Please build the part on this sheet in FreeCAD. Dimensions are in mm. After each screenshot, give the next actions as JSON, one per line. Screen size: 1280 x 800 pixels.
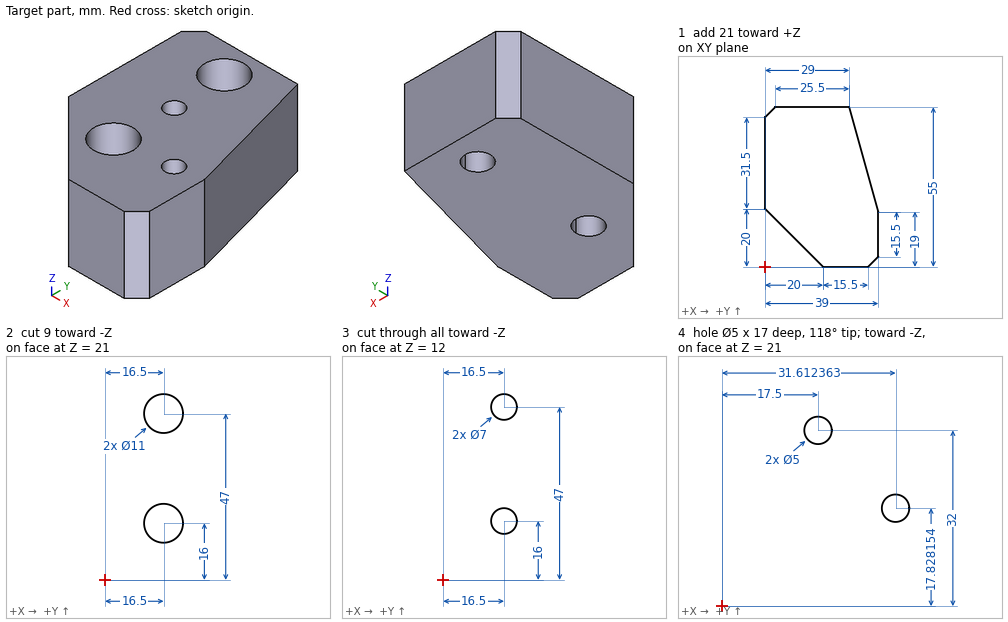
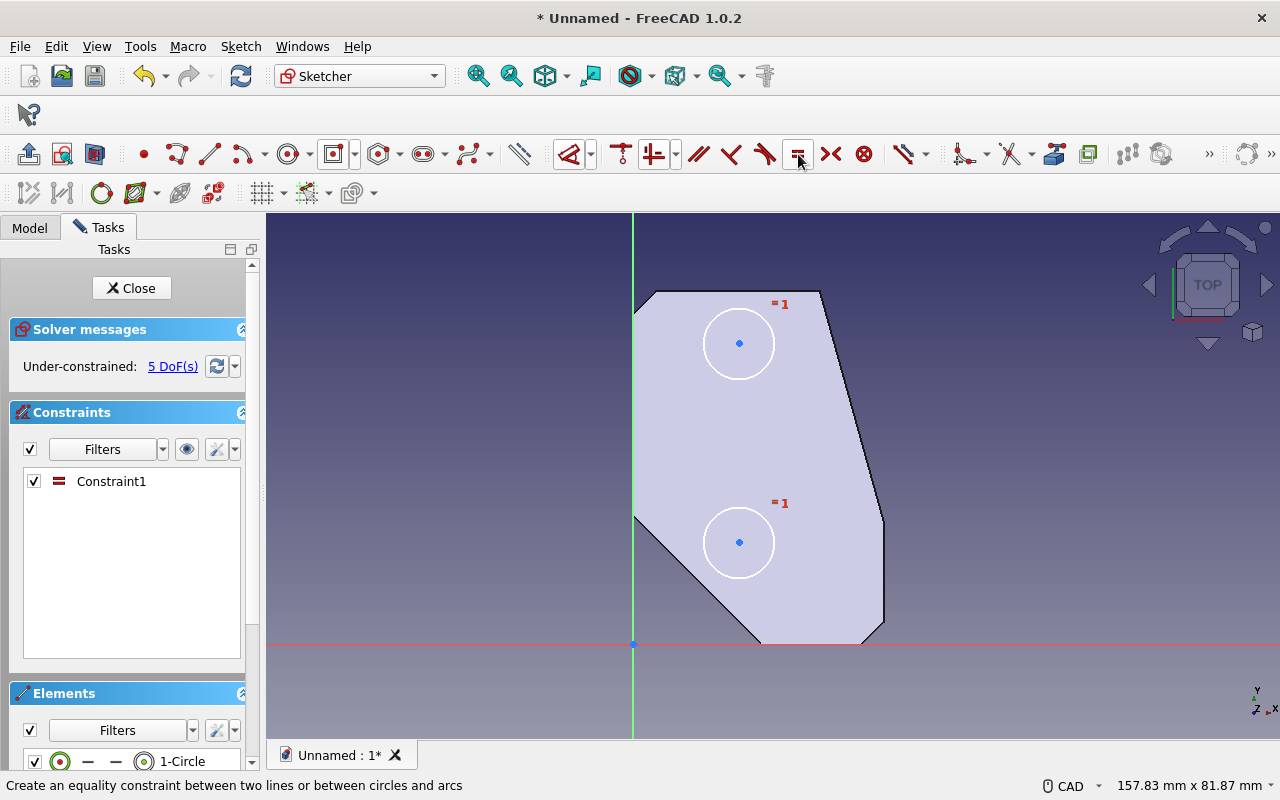
{"action": "left_click", "coordinate": [764, 319]}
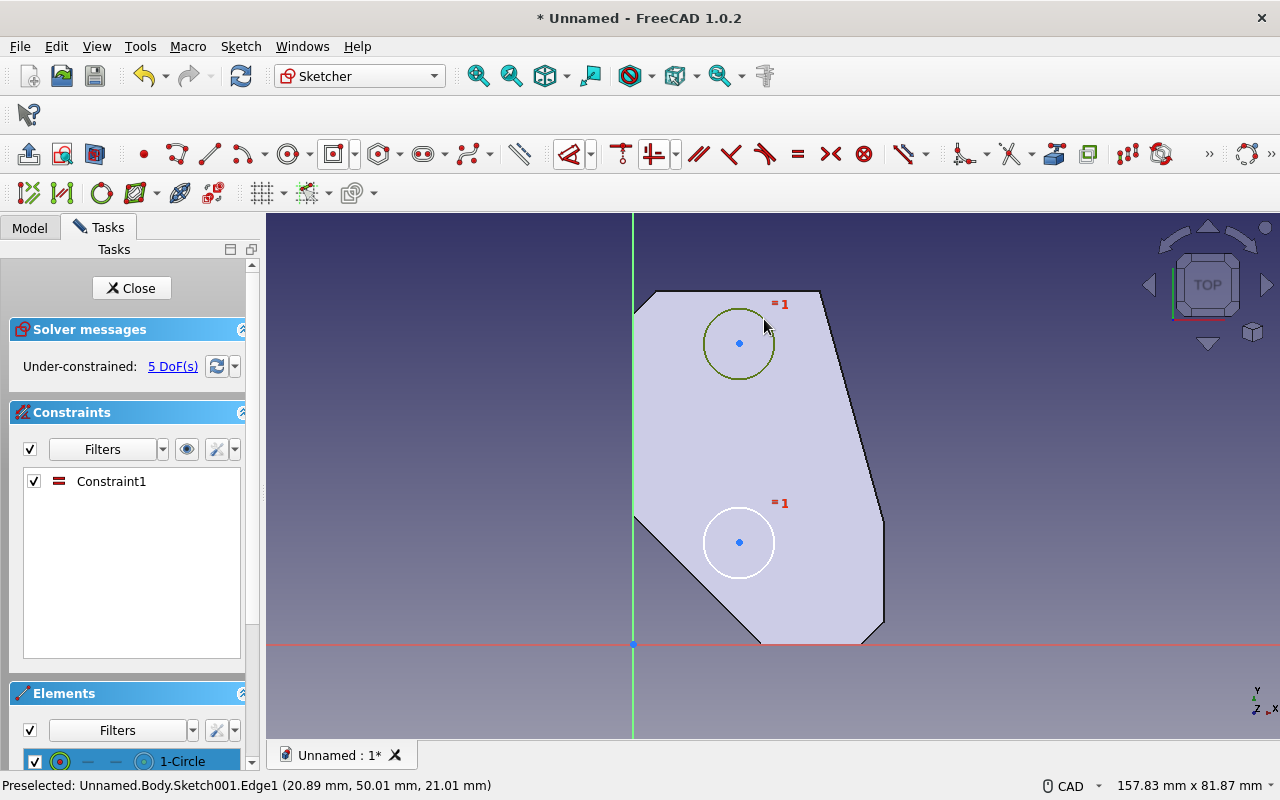
{"action": "left_click", "coordinate": [590, 154]}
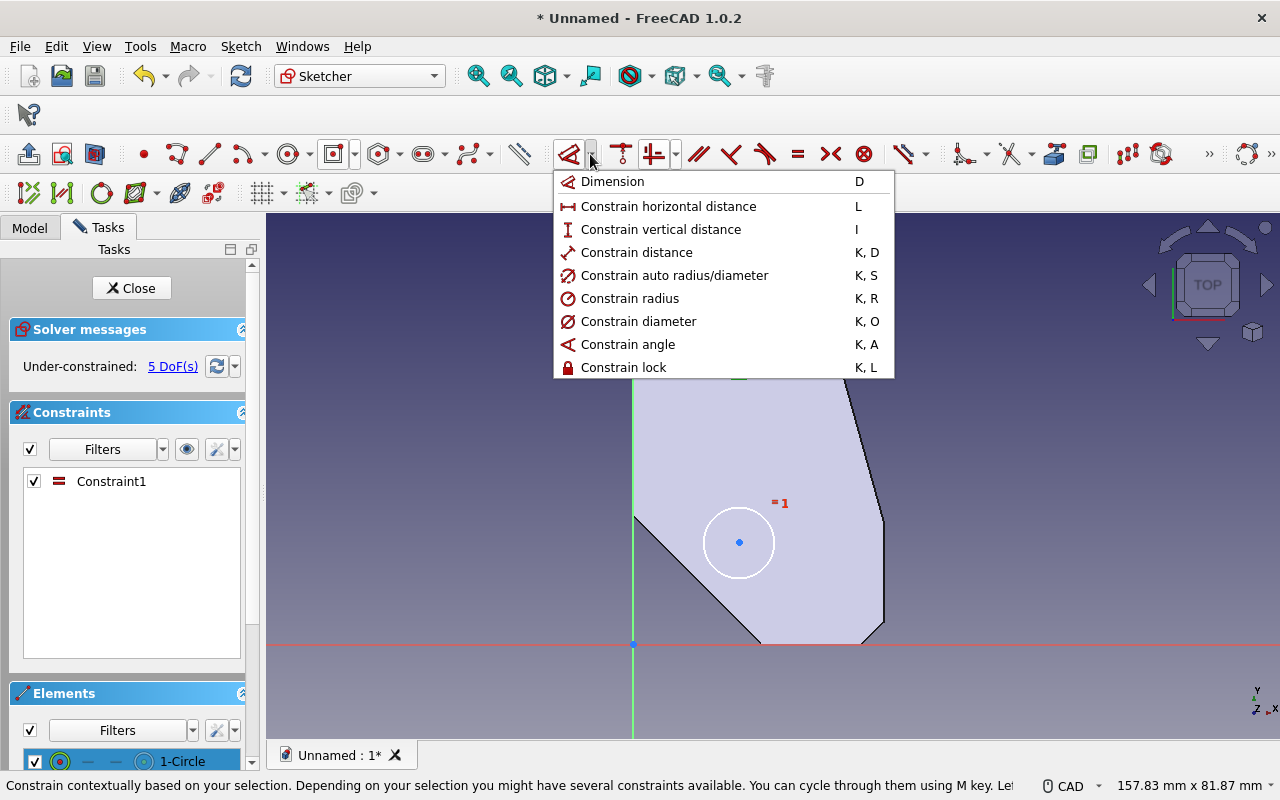
{"action": "left_click", "coordinate": [724, 322]}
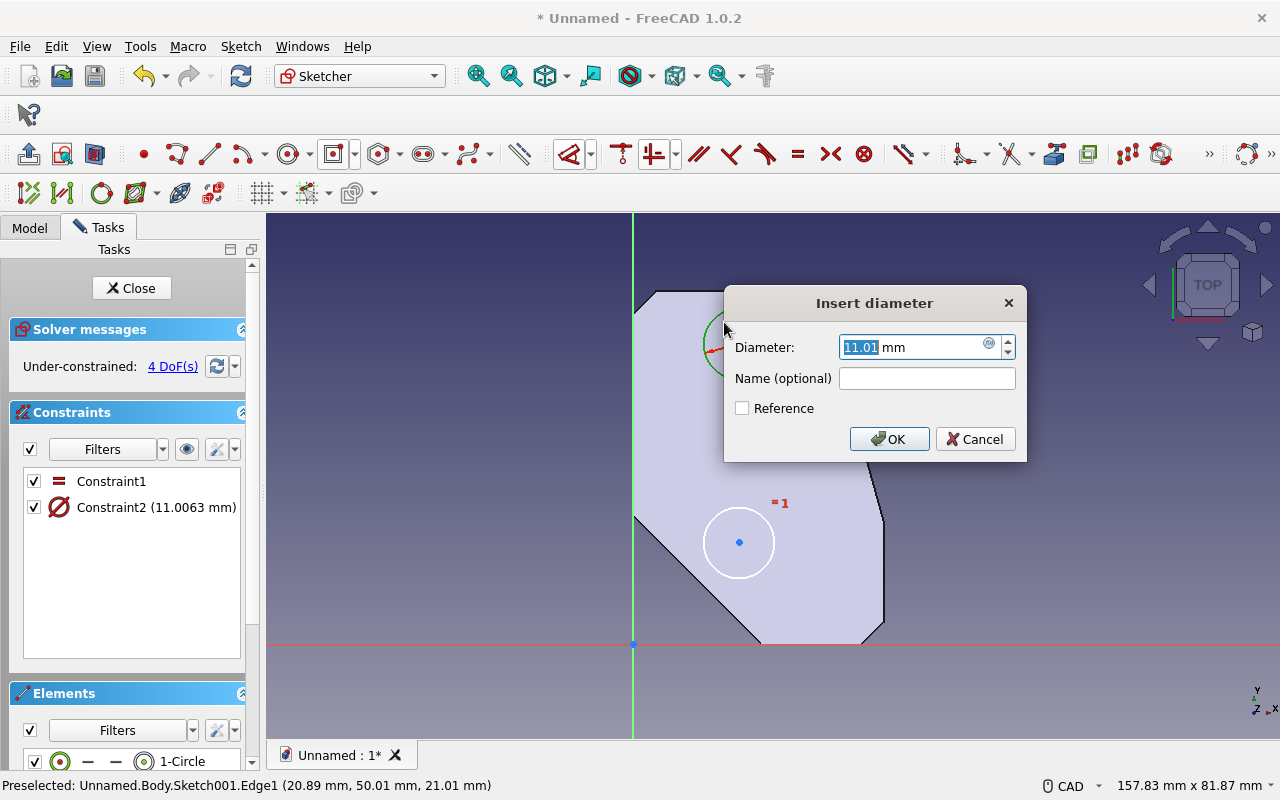
{"action": "type", "text": "11"}
{"action": "key", "text": "Return"}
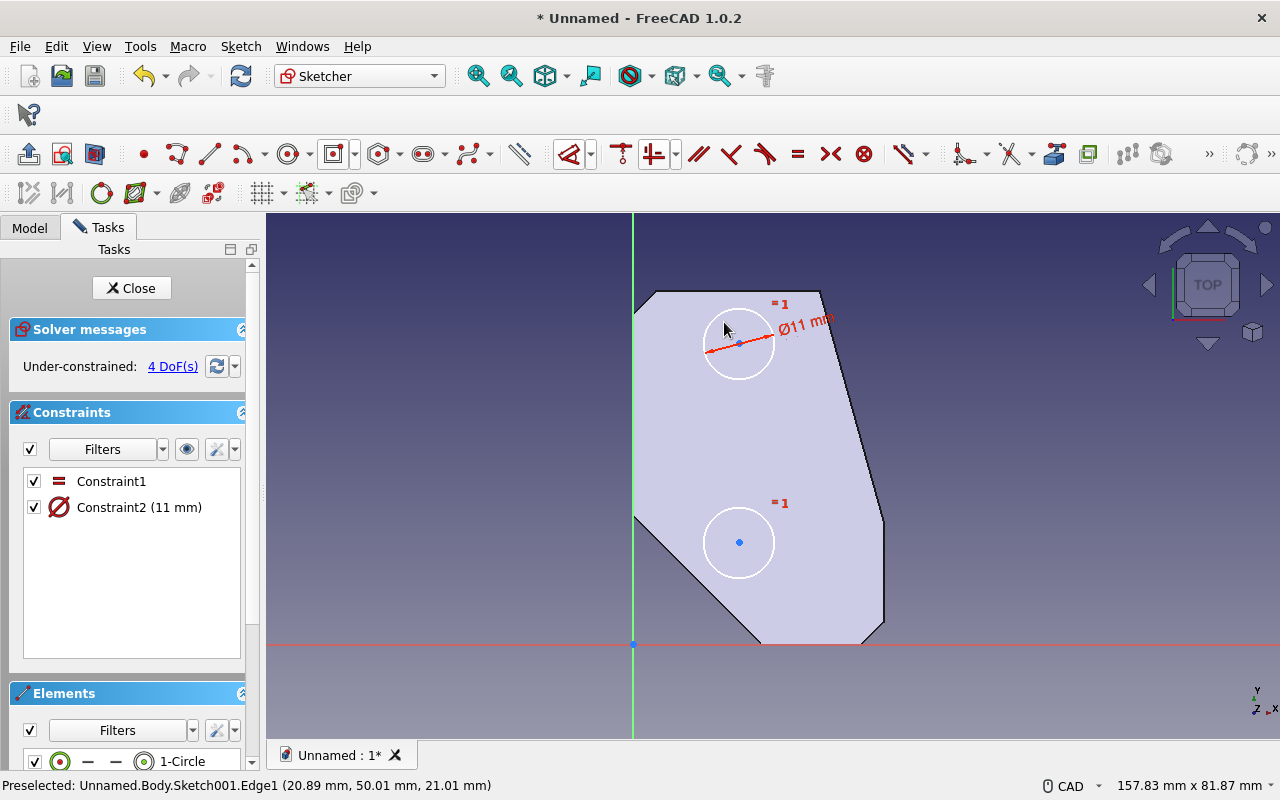
{"action": "left_click", "coordinate": [739, 344]}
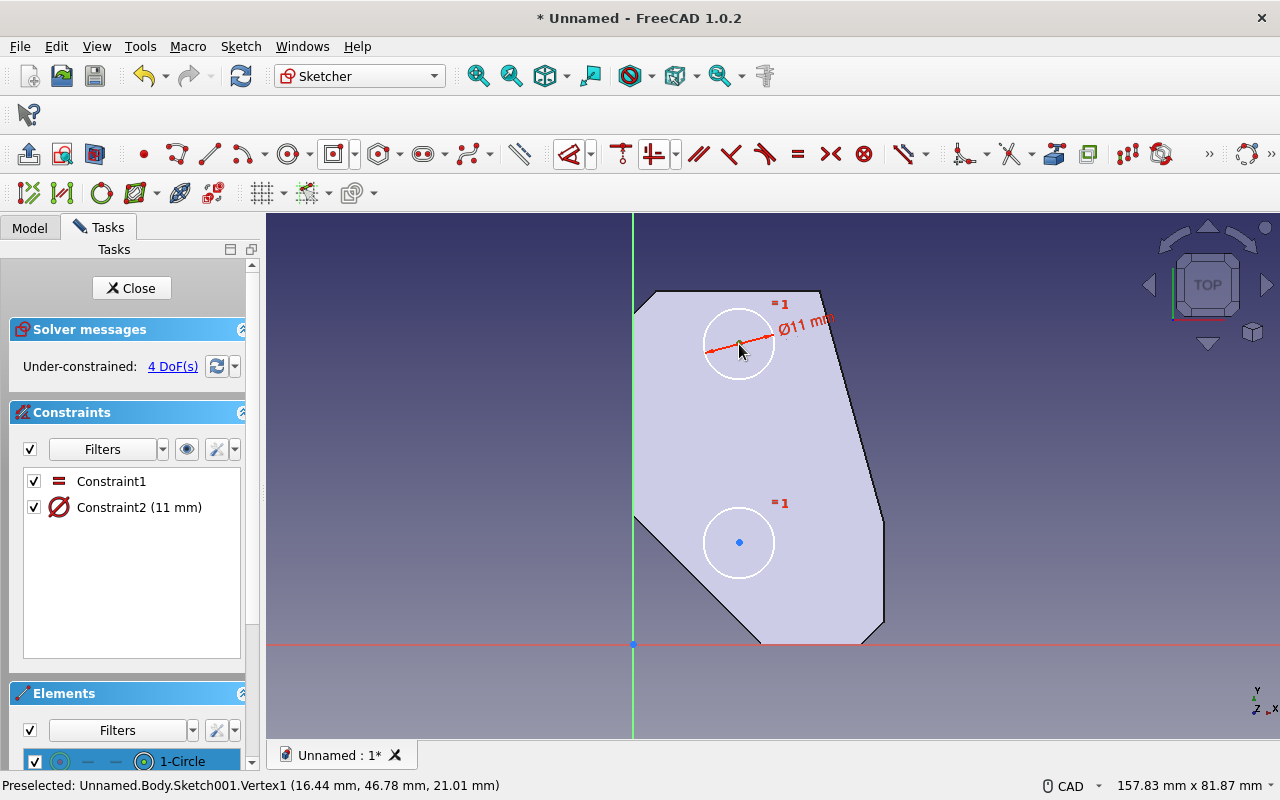
{"action": "left_click", "coordinate": [590, 154]}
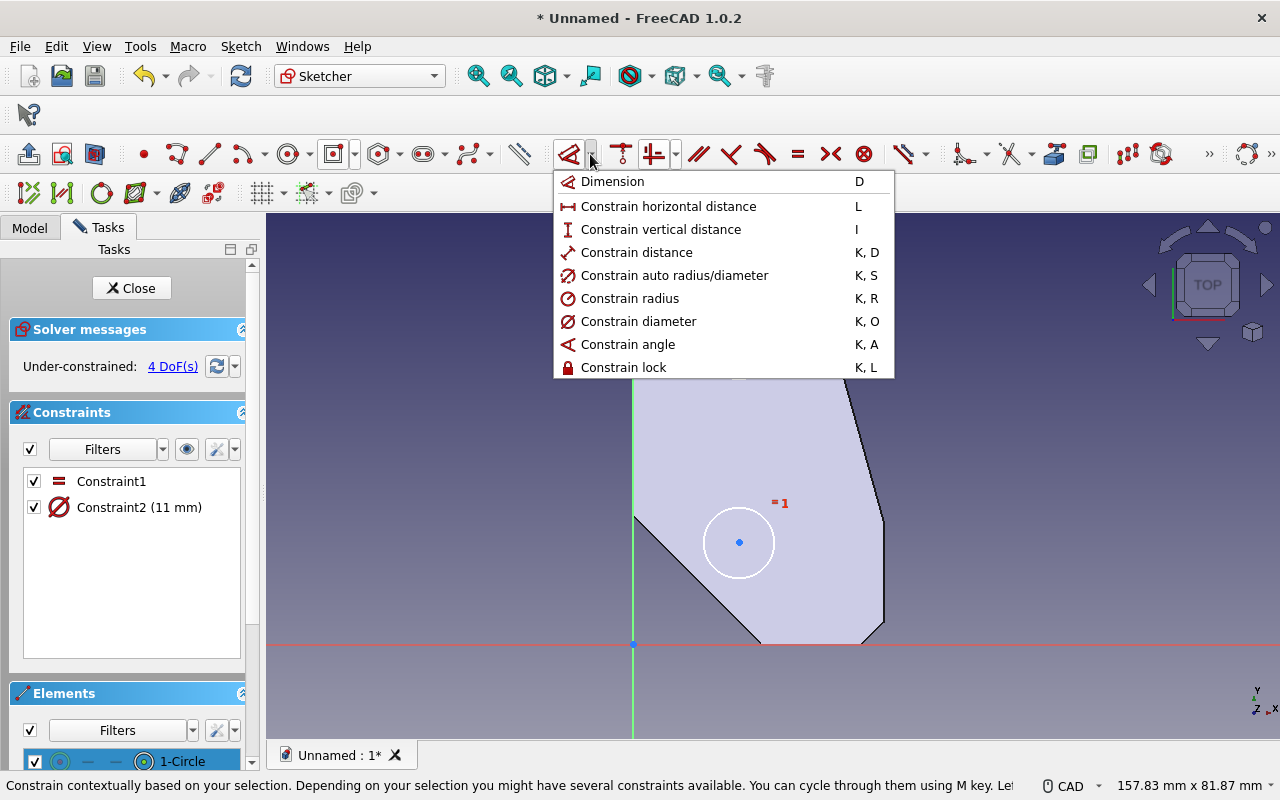
{"action": "left_click", "coordinate": [724, 230]}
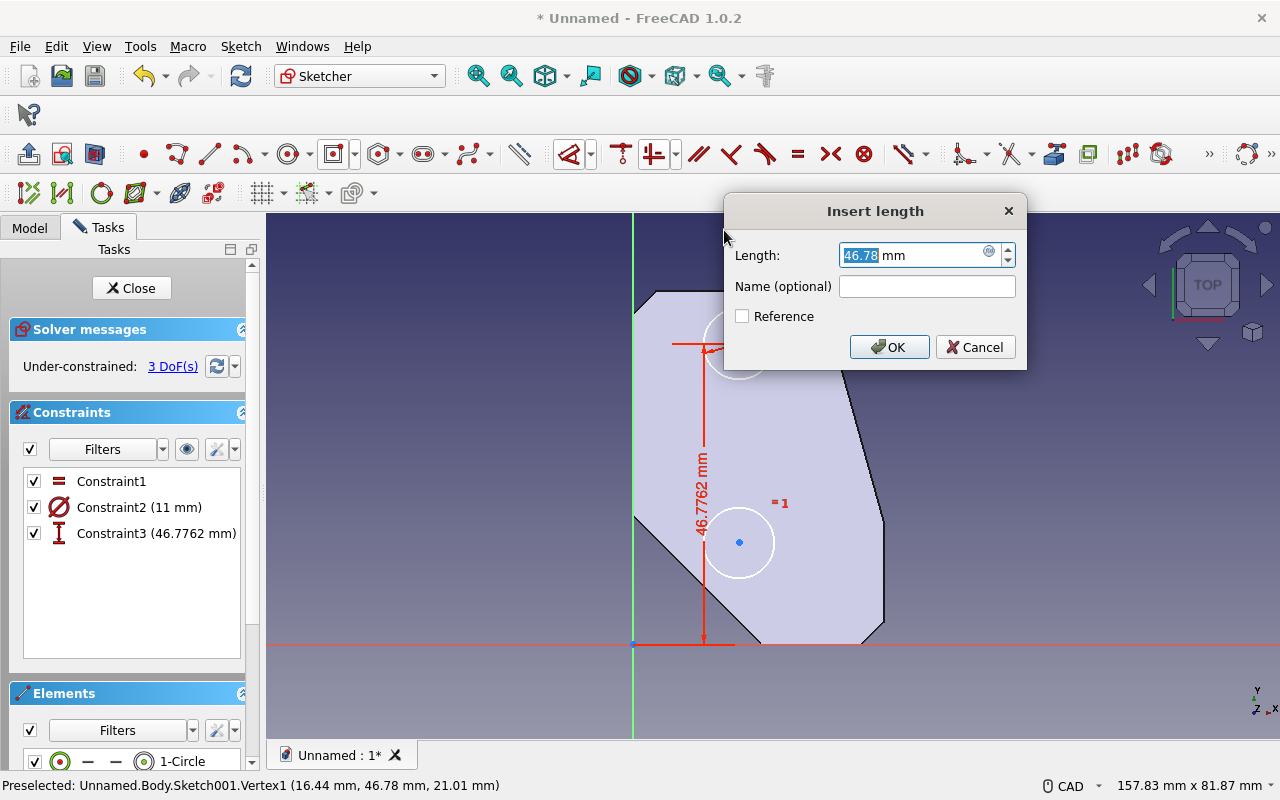
{"action": "type", "text": "47"}
{"action": "key", "text": "Return"}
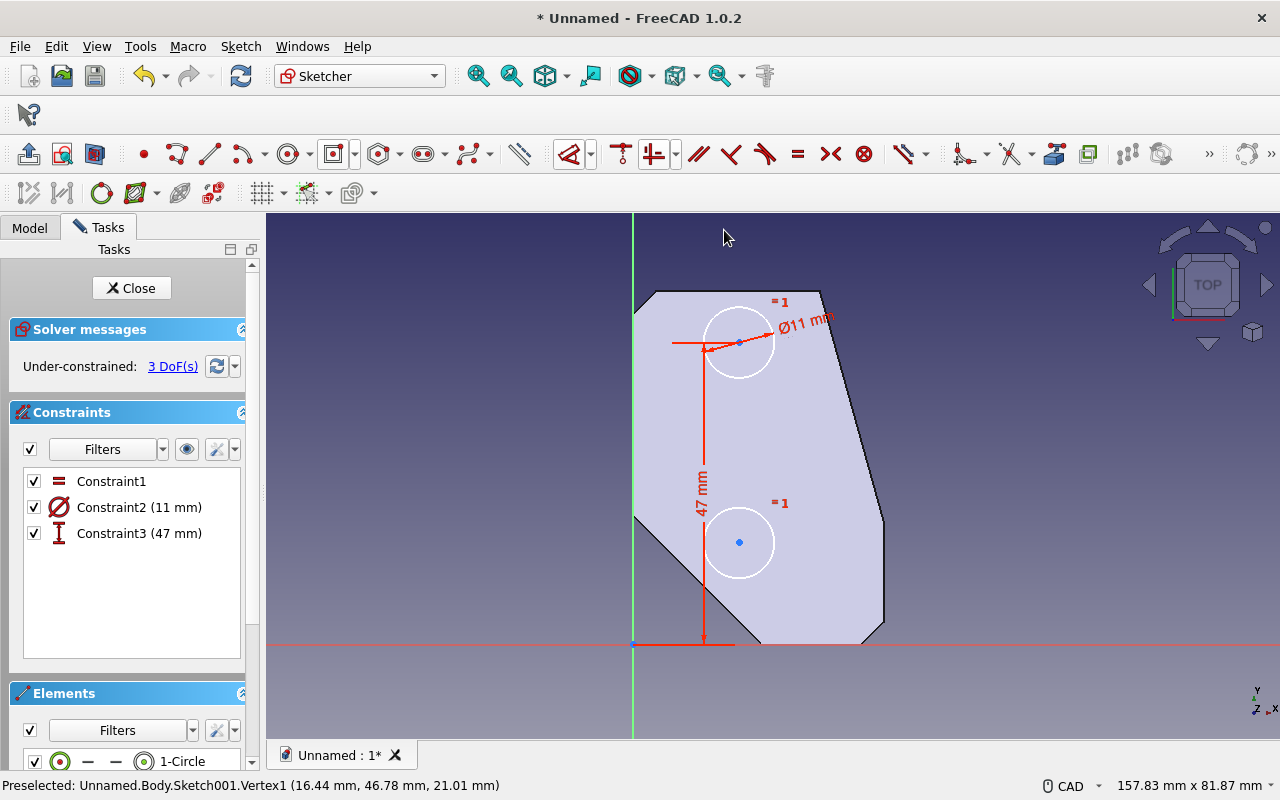
{"action": "left_click", "coordinate": [739, 543]}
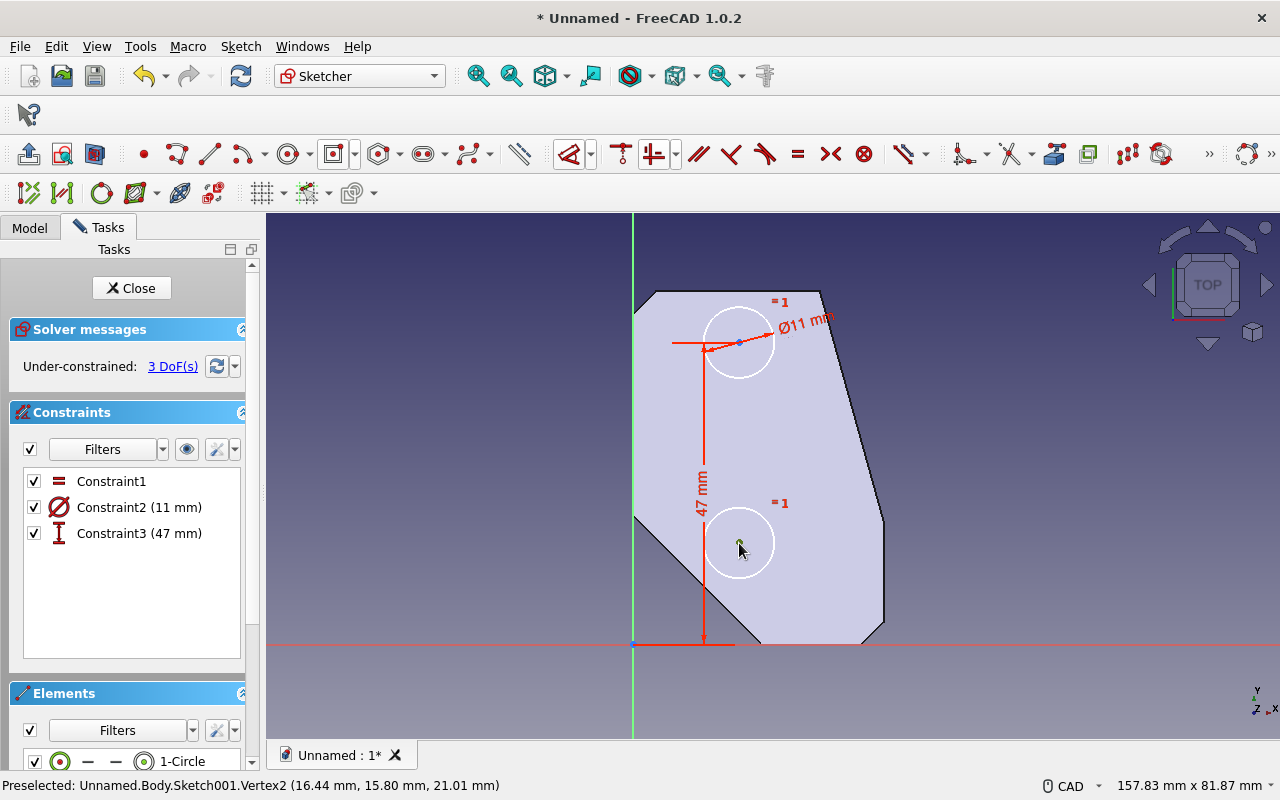
{"action": "left_click", "coordinate": [590, 154]}